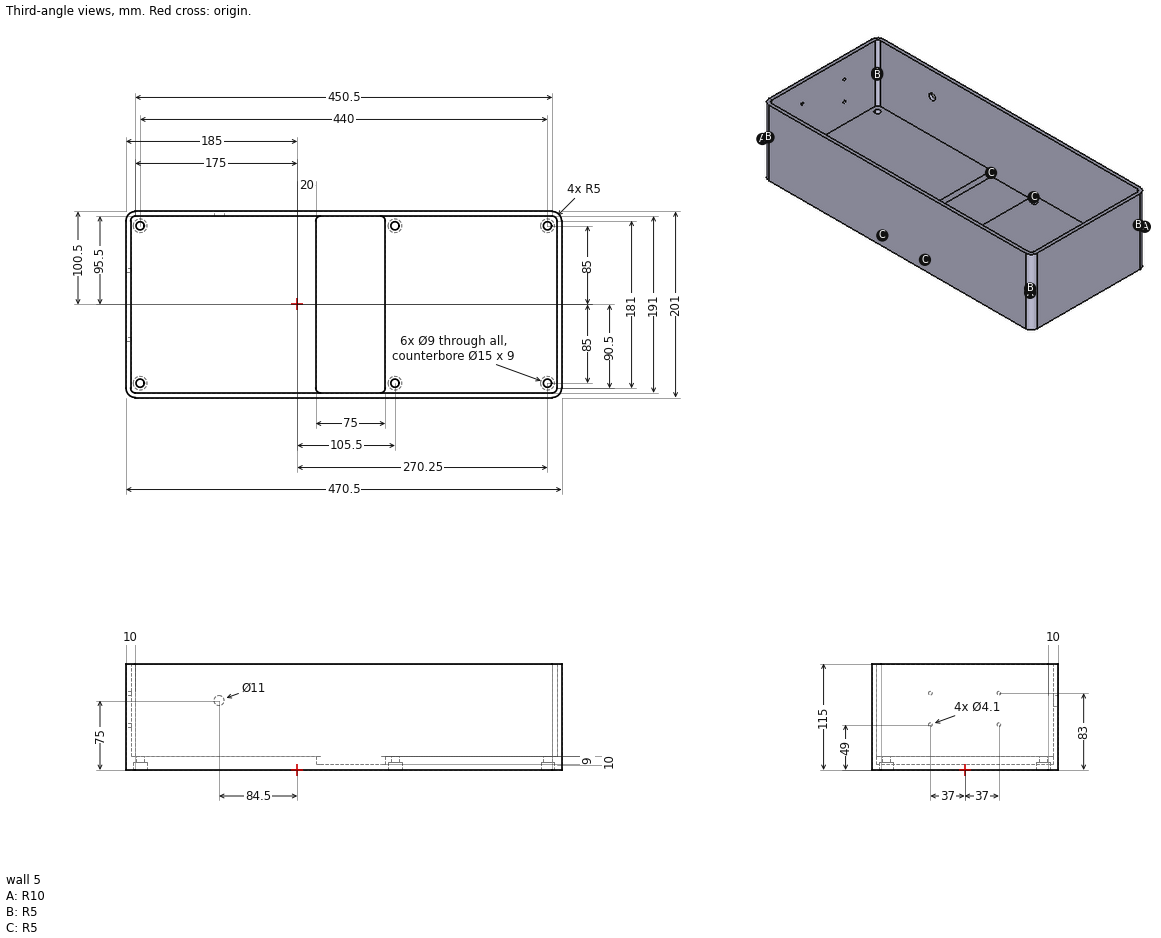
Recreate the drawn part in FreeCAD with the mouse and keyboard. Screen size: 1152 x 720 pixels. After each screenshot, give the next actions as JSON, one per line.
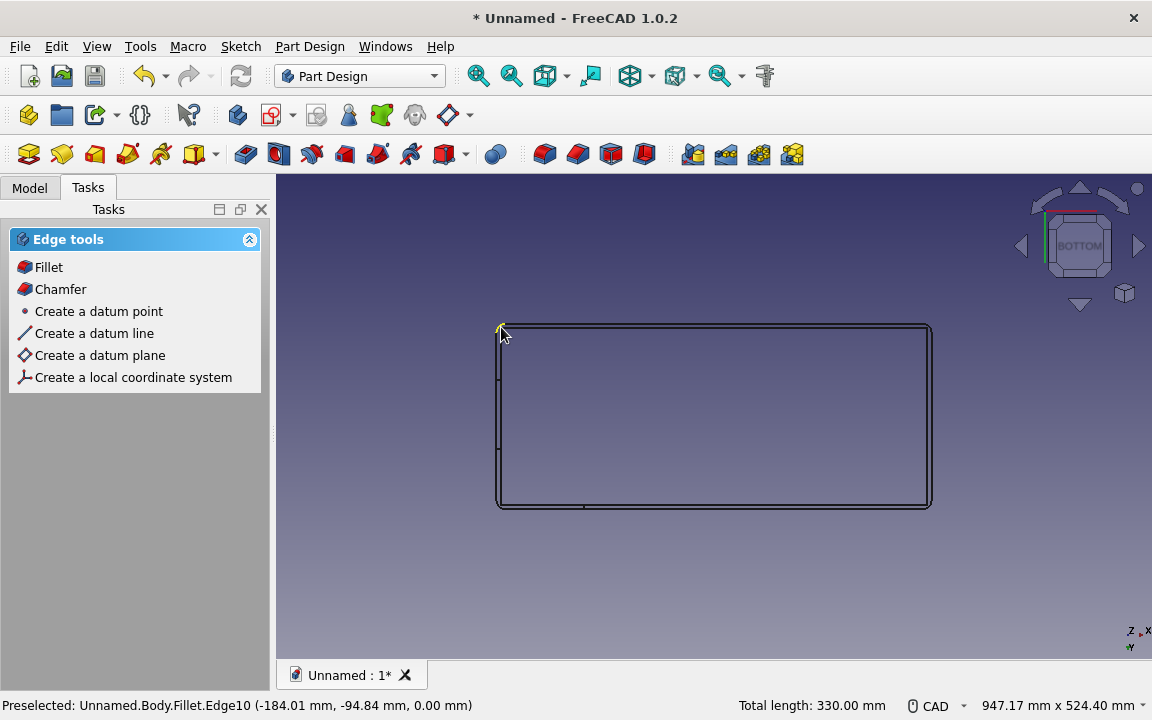
{"action": "key", "text": "4"}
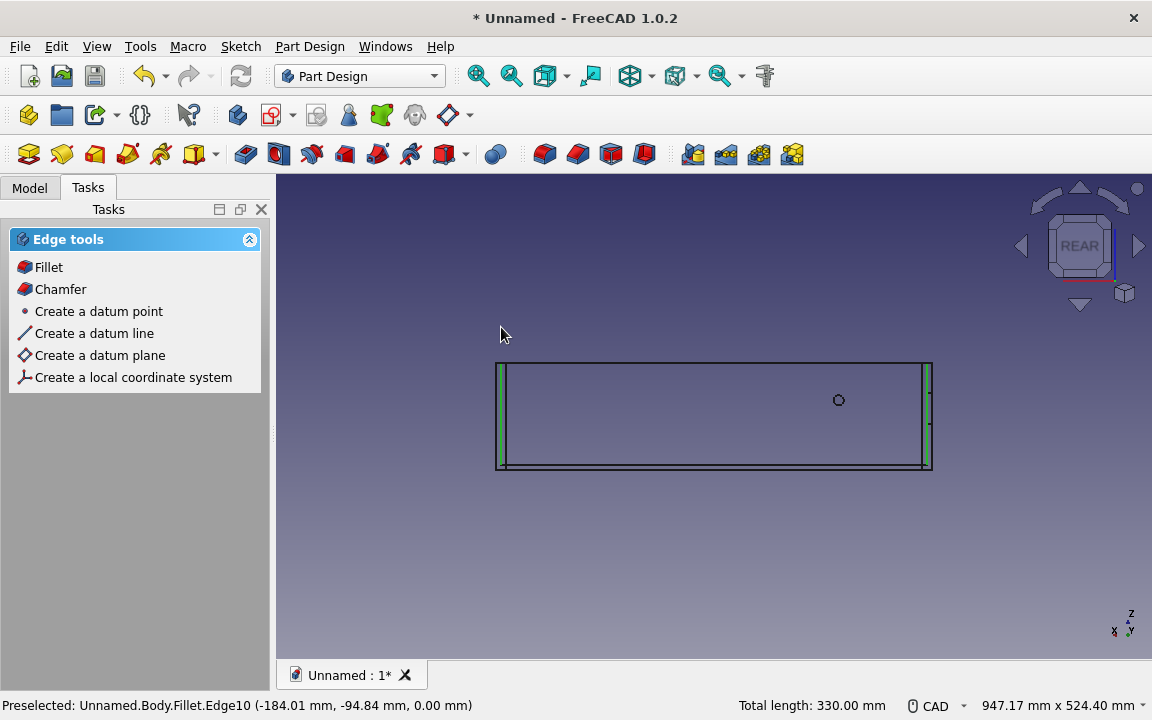
{"action": "scroll", "coordinate": [927, 413], "scroll_direction": "up", "scroll_amount": 6}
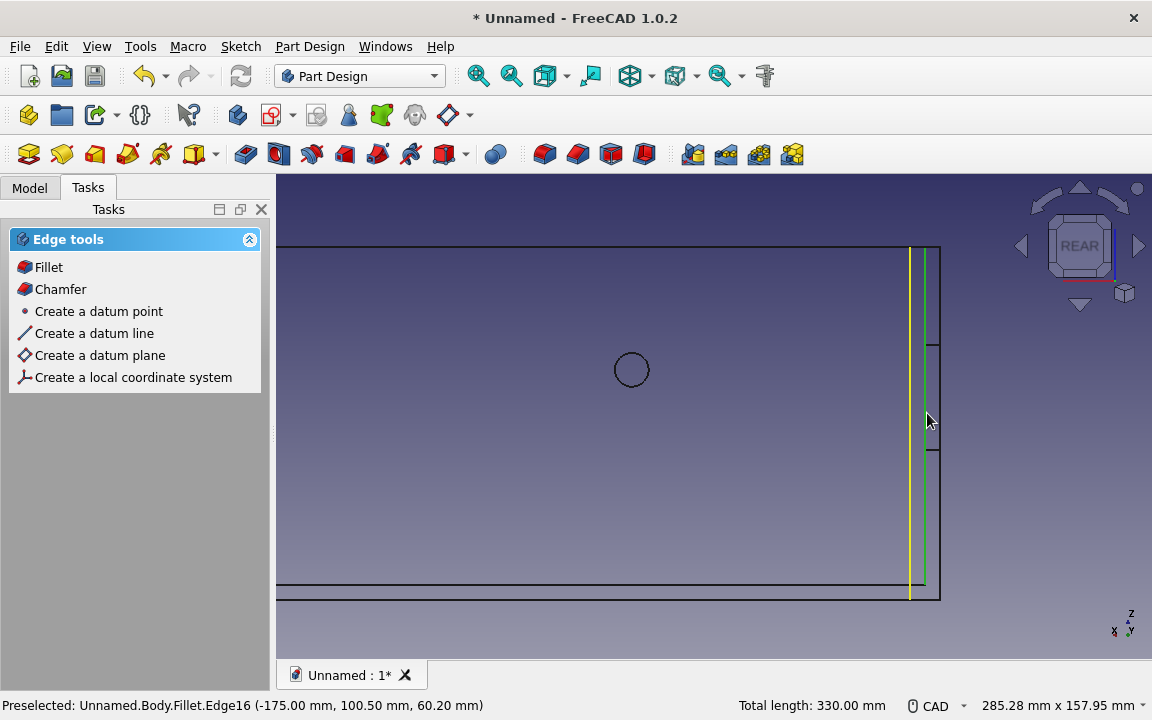
{"action": "left_click", "coordinate": [479, 76]}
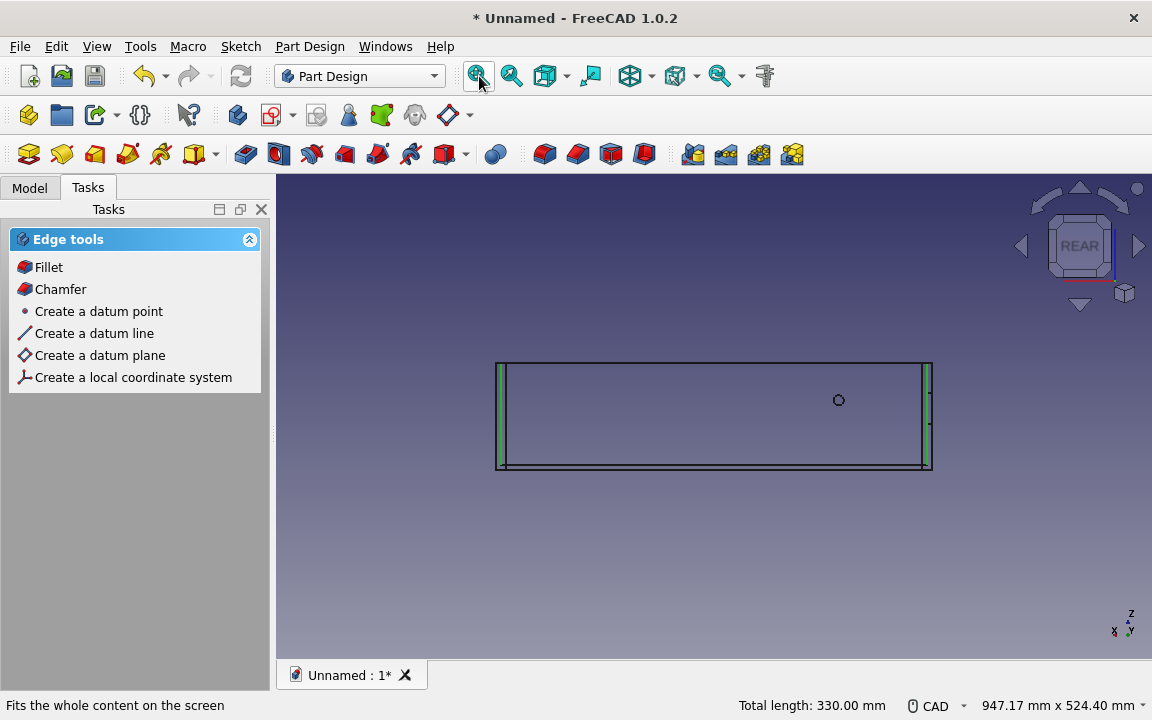
{"action": "key", "text": "6"}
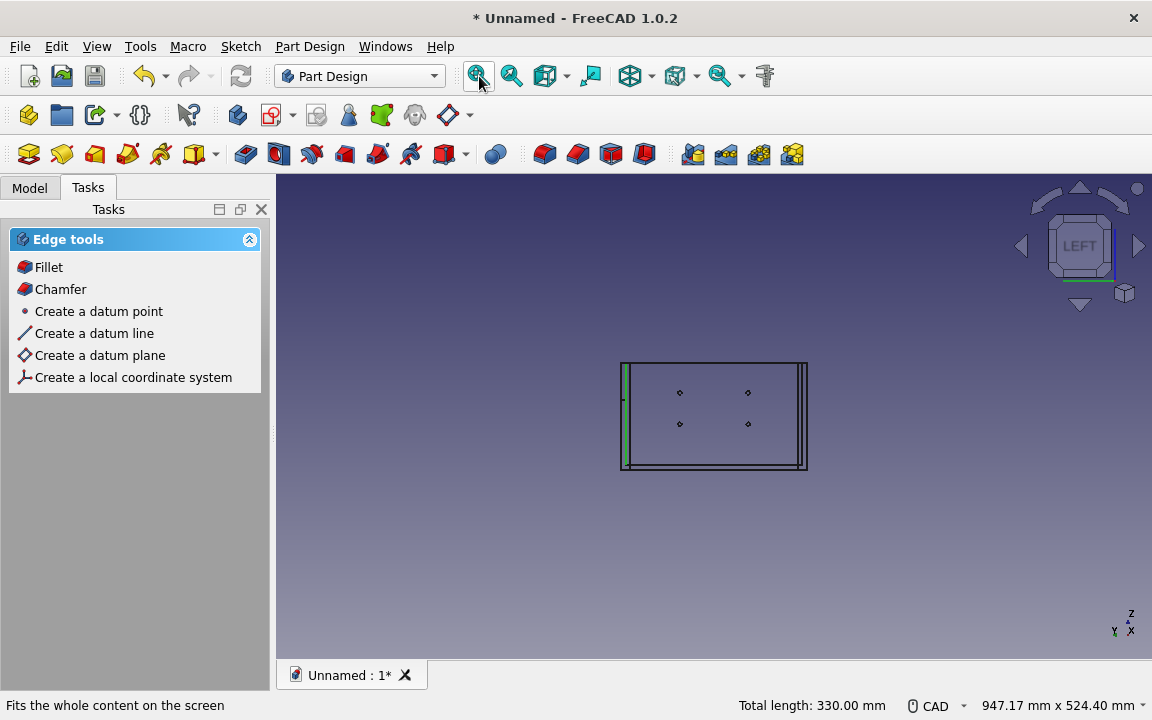
{"action": "key", "text": "v f"}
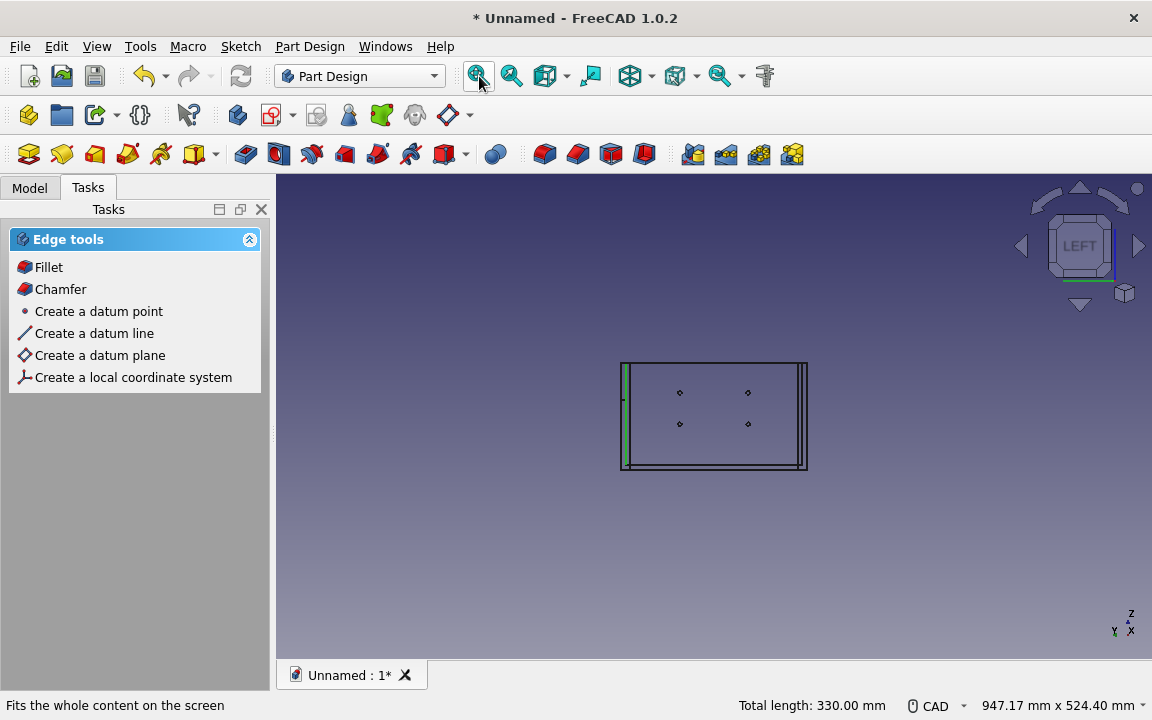
{"action": "scroll", "coordinate": [802, 413], "scroll_direction": "up", "scroll_amount": 6}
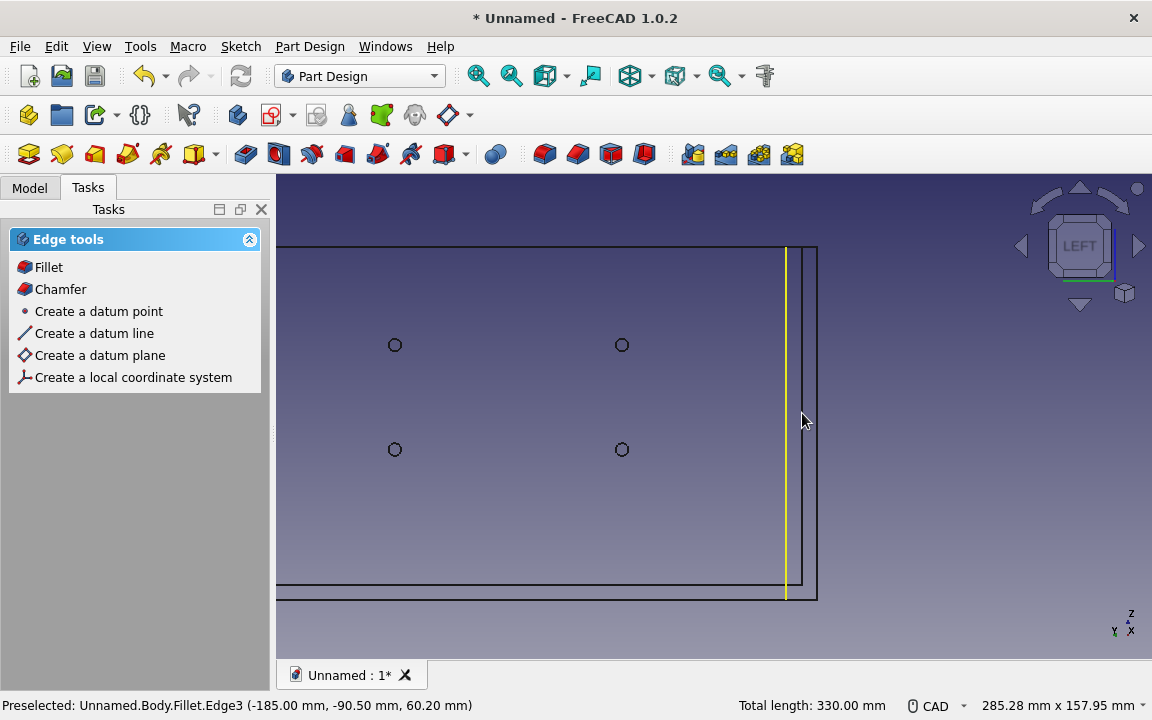
{"action": "left_click", "coordinate": [802, 415], "text": "ctrl"}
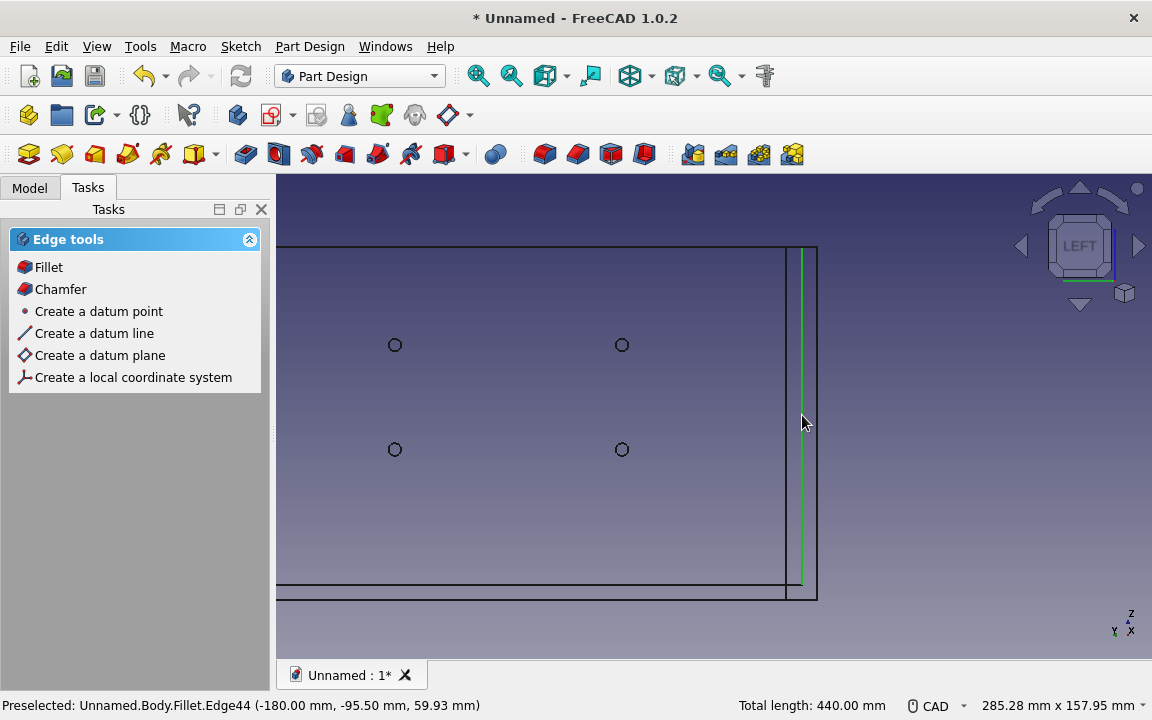
{"action": "key", "text": "v 1"}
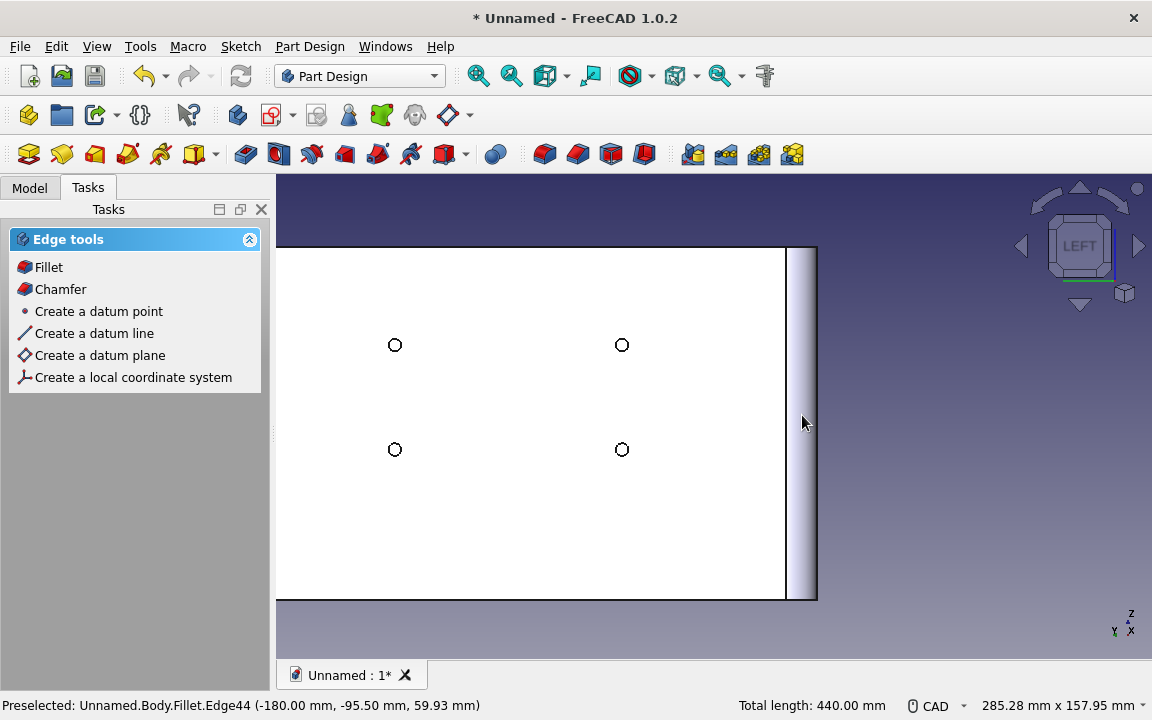
{"action": "left_click", "coordinate": [545, 154]}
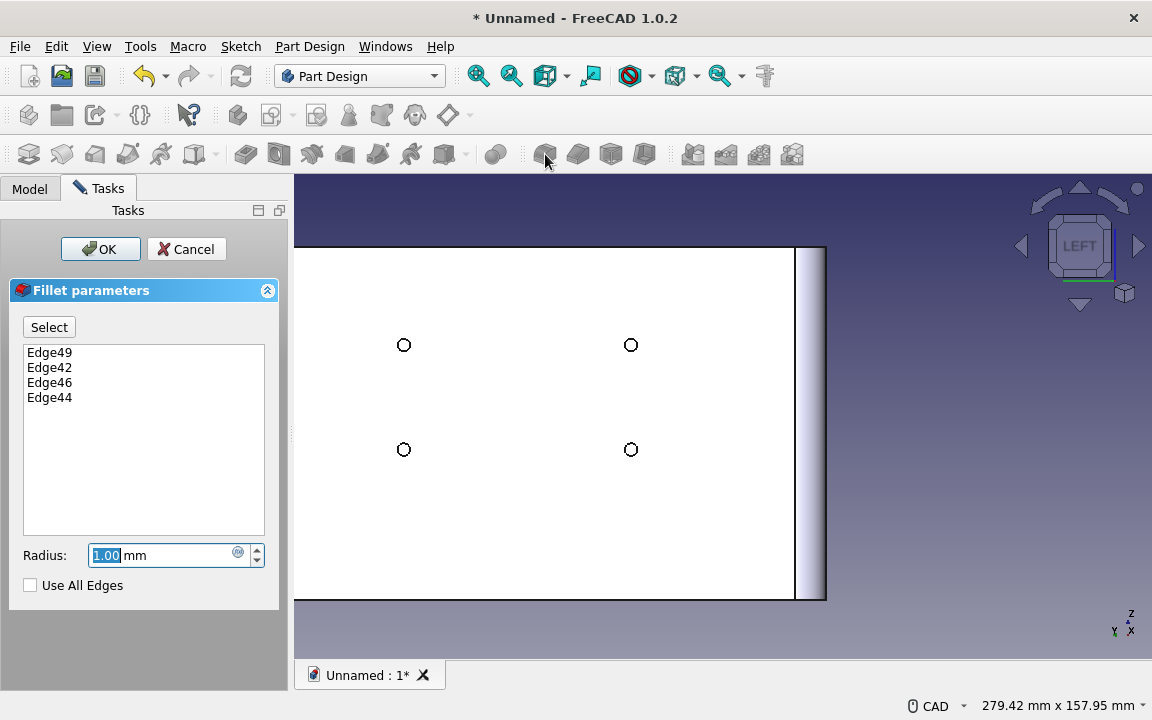
{"action": "type", "text": "5"}
{"action": "key", "text": "Tab"}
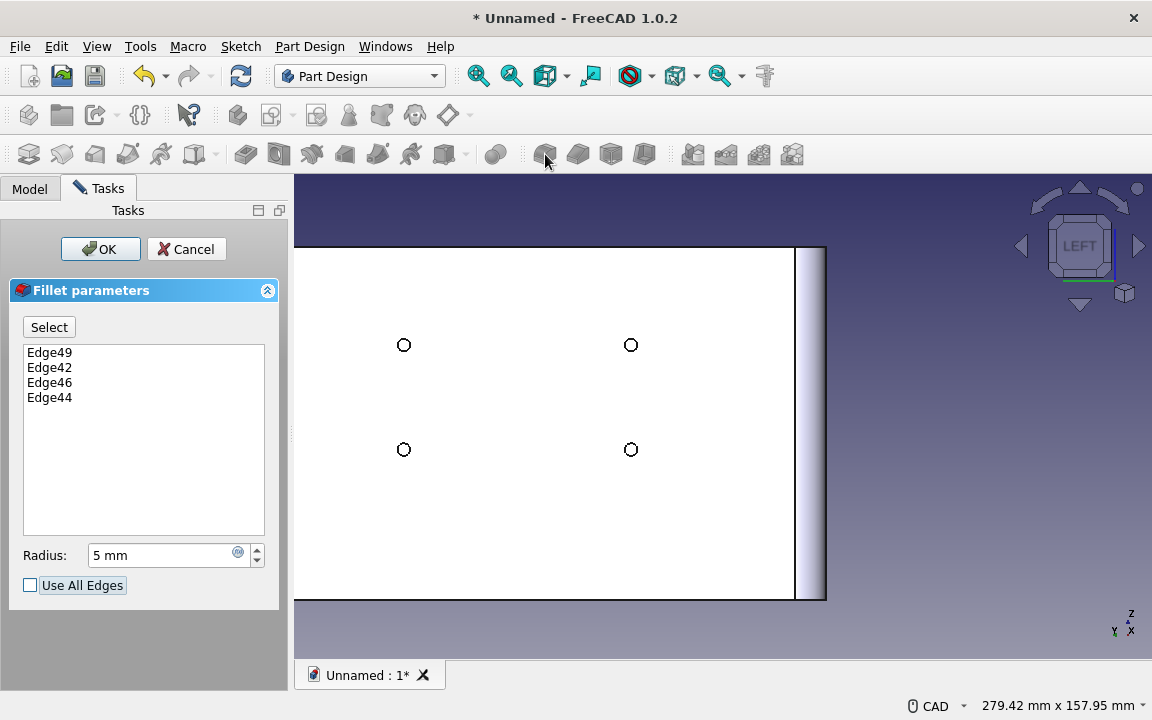
{"action": "left_click", "coordinate": [101, 249]}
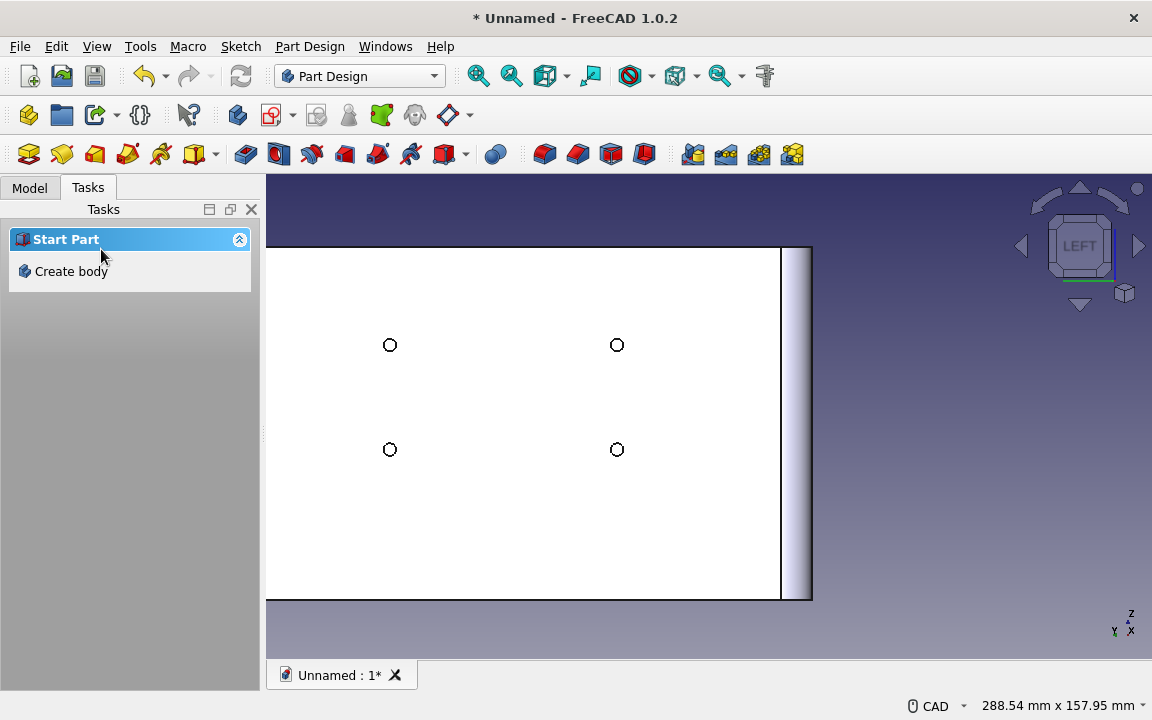
{"action": "key", "text": "v f"}